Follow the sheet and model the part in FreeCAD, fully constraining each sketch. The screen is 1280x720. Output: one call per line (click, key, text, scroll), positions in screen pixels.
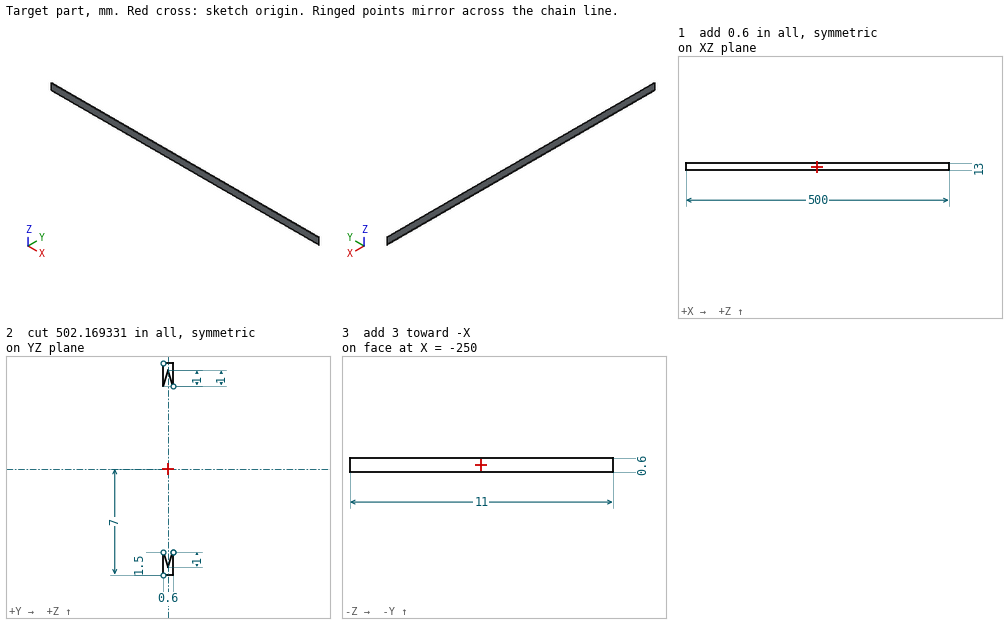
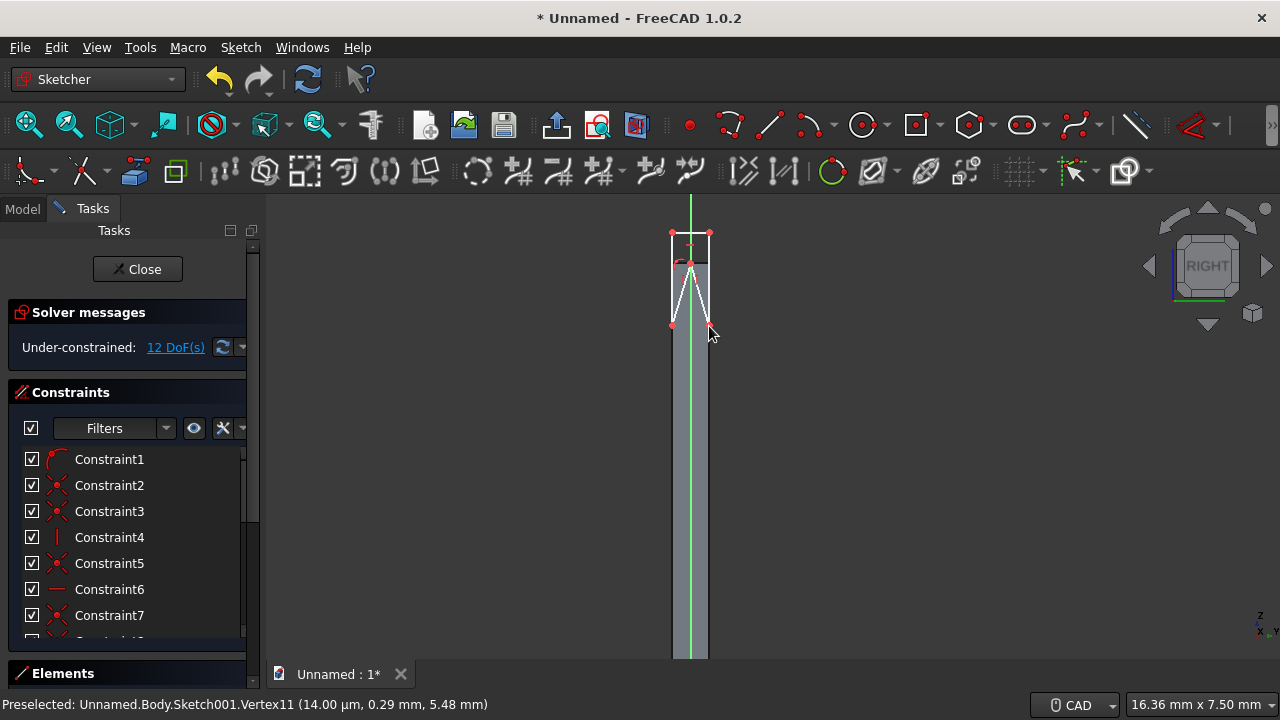
scroll(710, 323, down, 6)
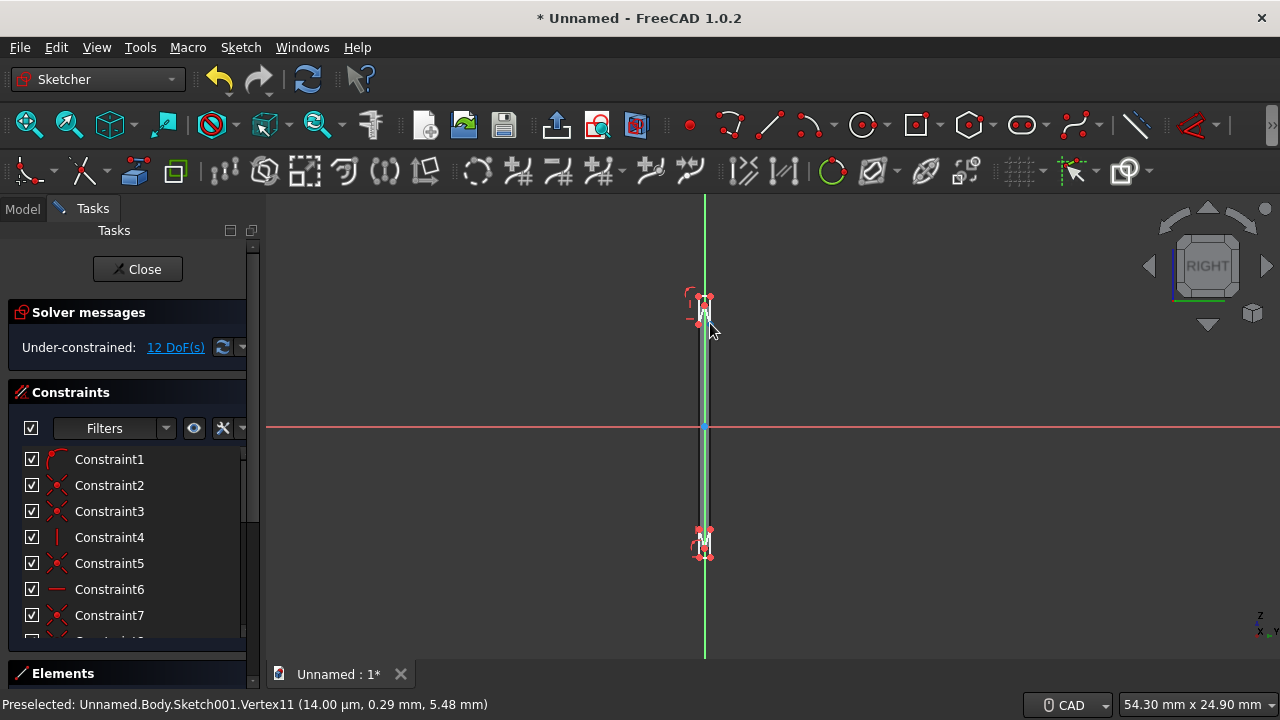
click(710, 530)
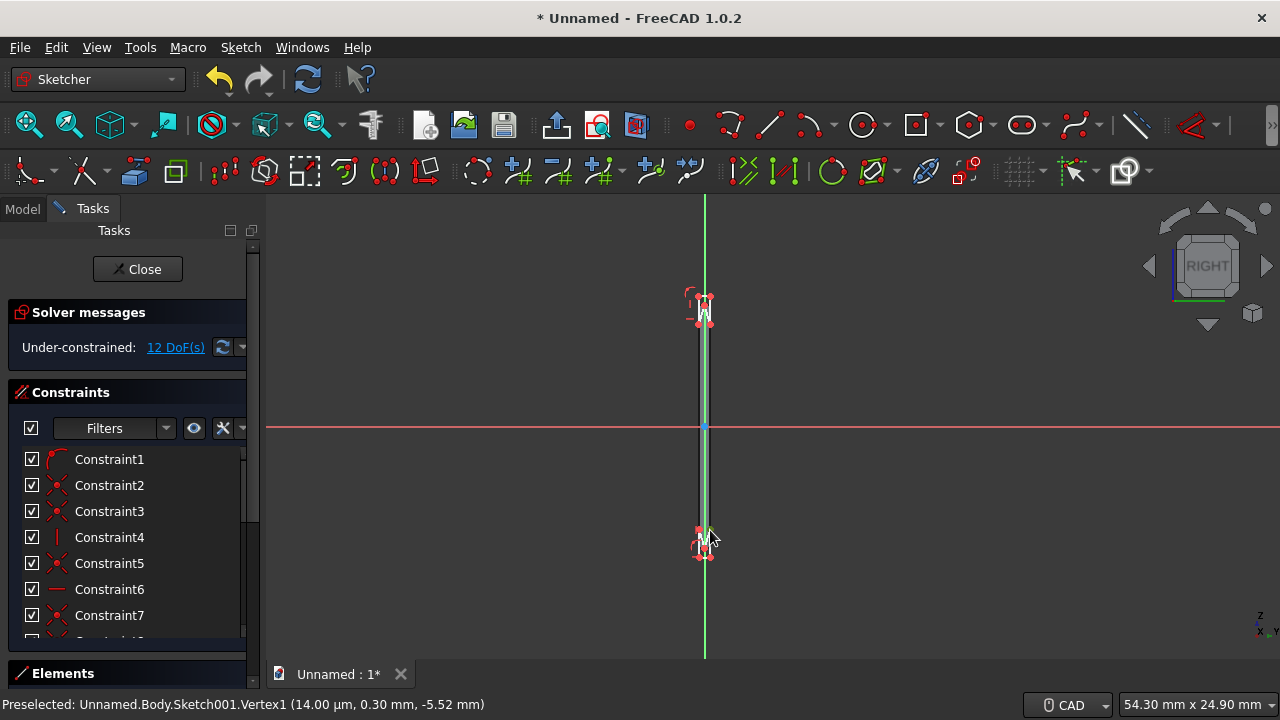
click(699, 530)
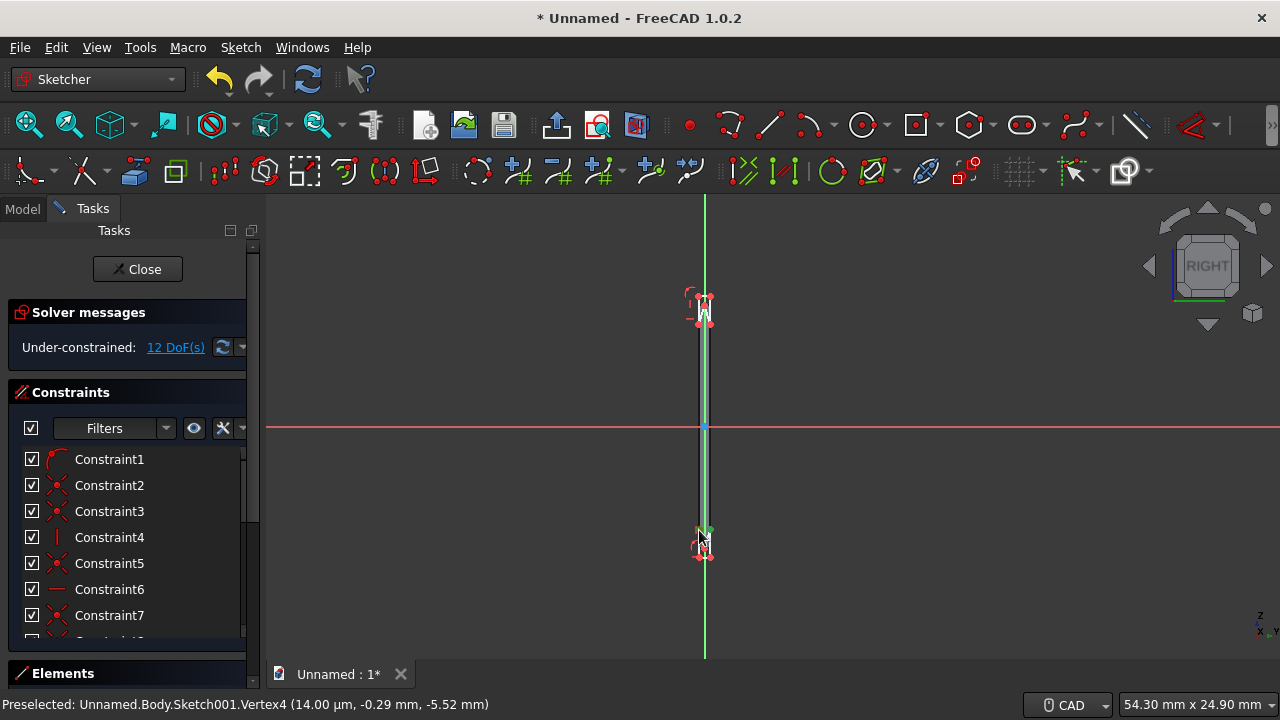
click(705, 602)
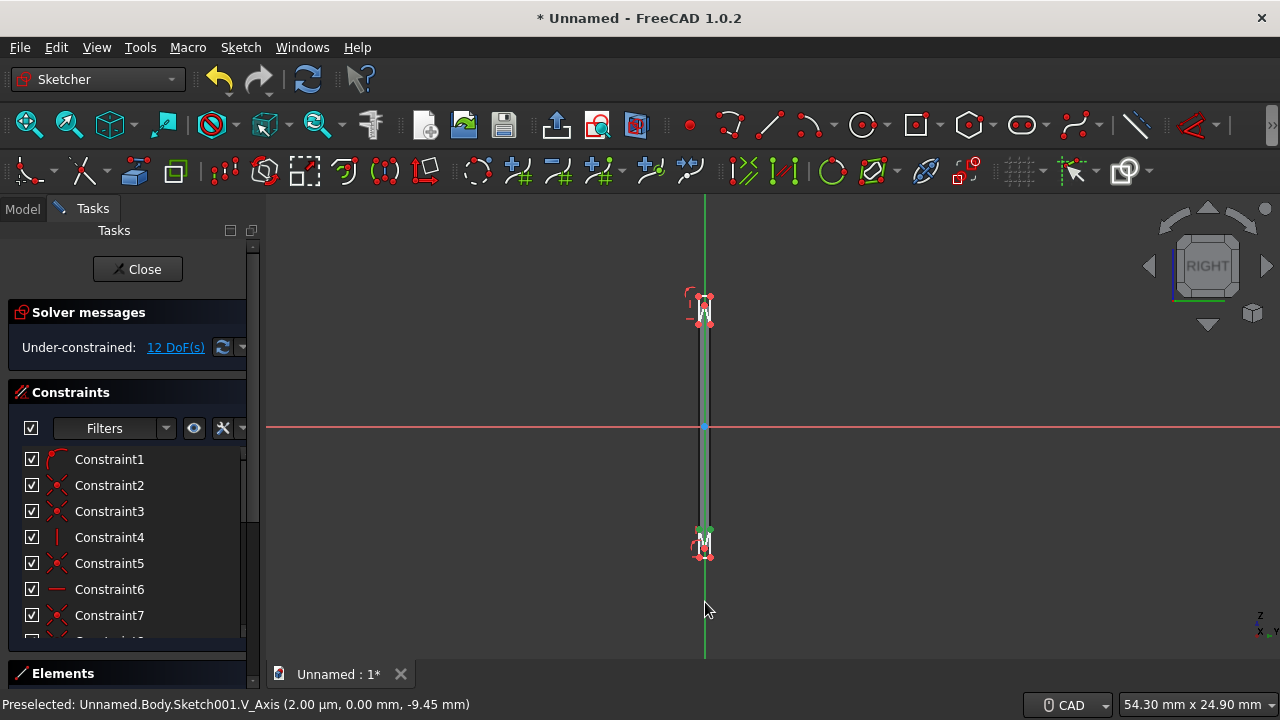
key(s)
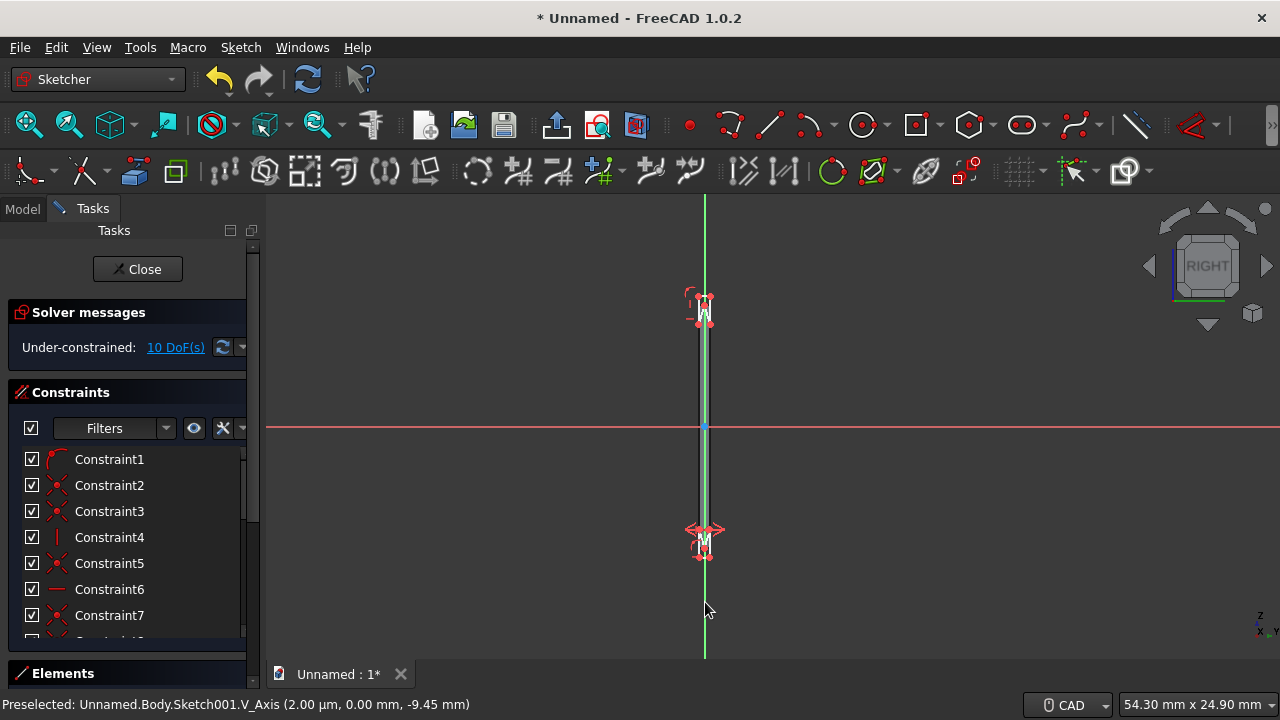
click(710, 530)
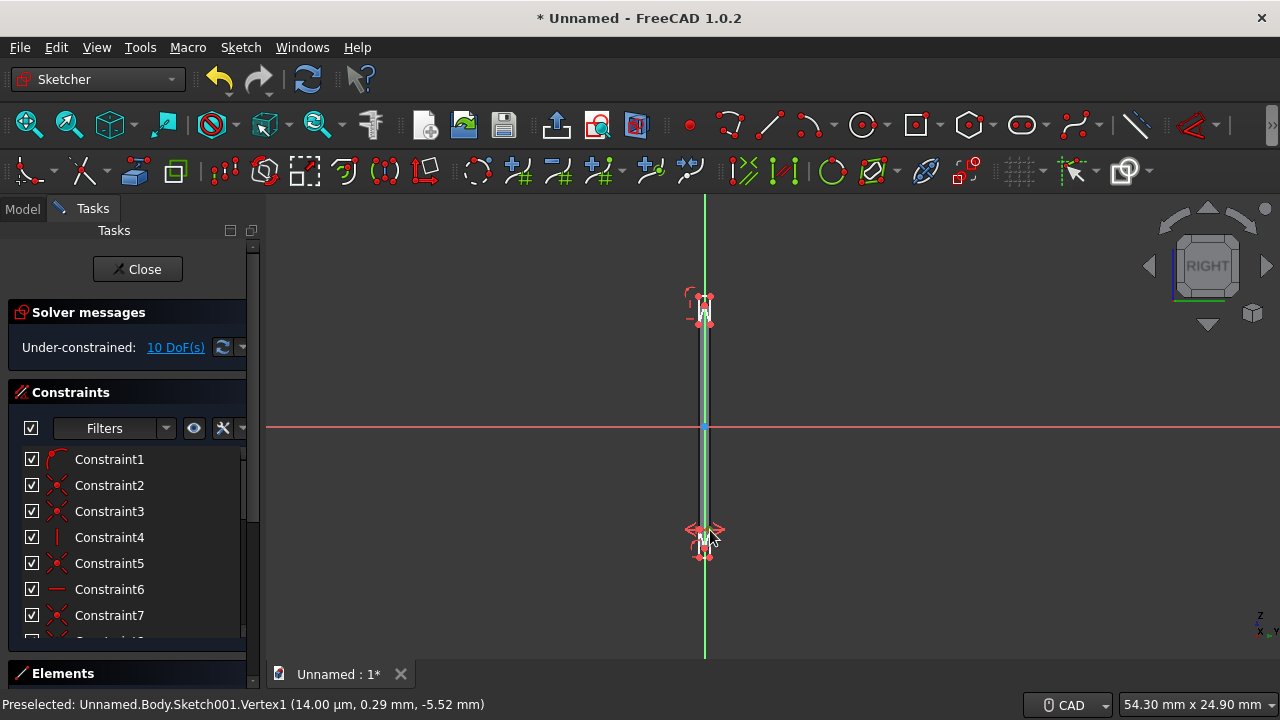
click(710, 324)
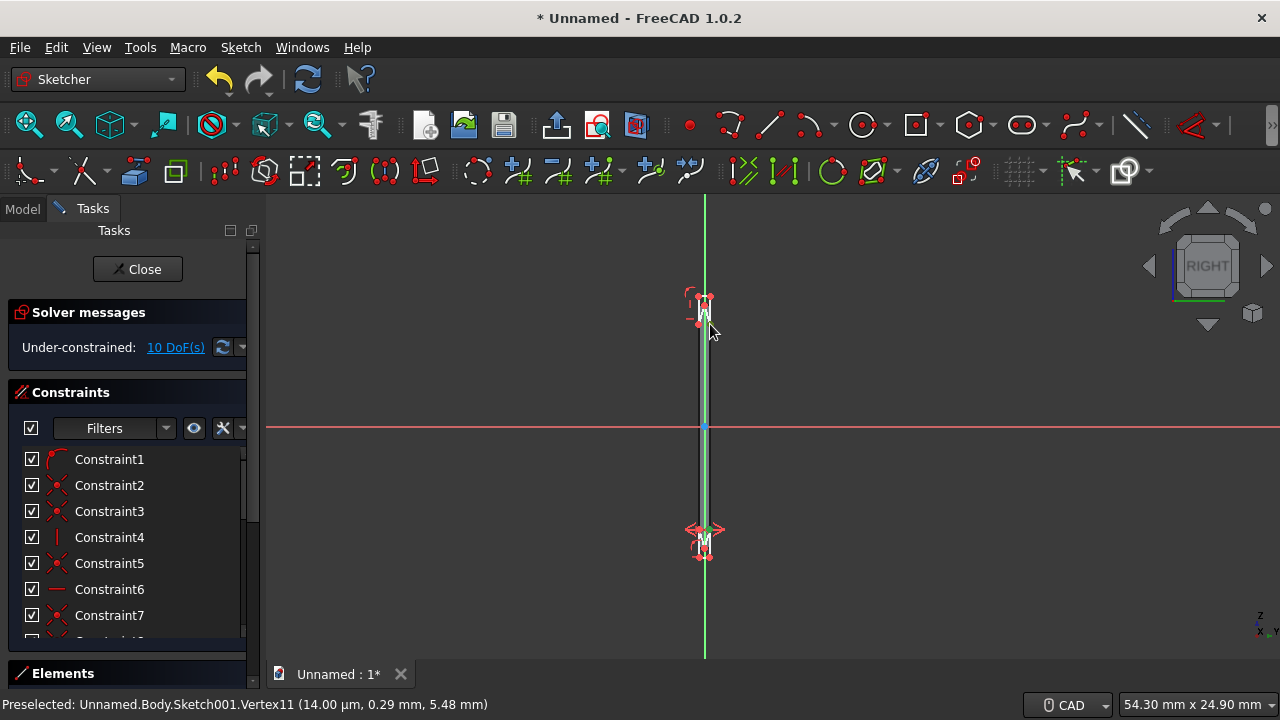
click(353, 426)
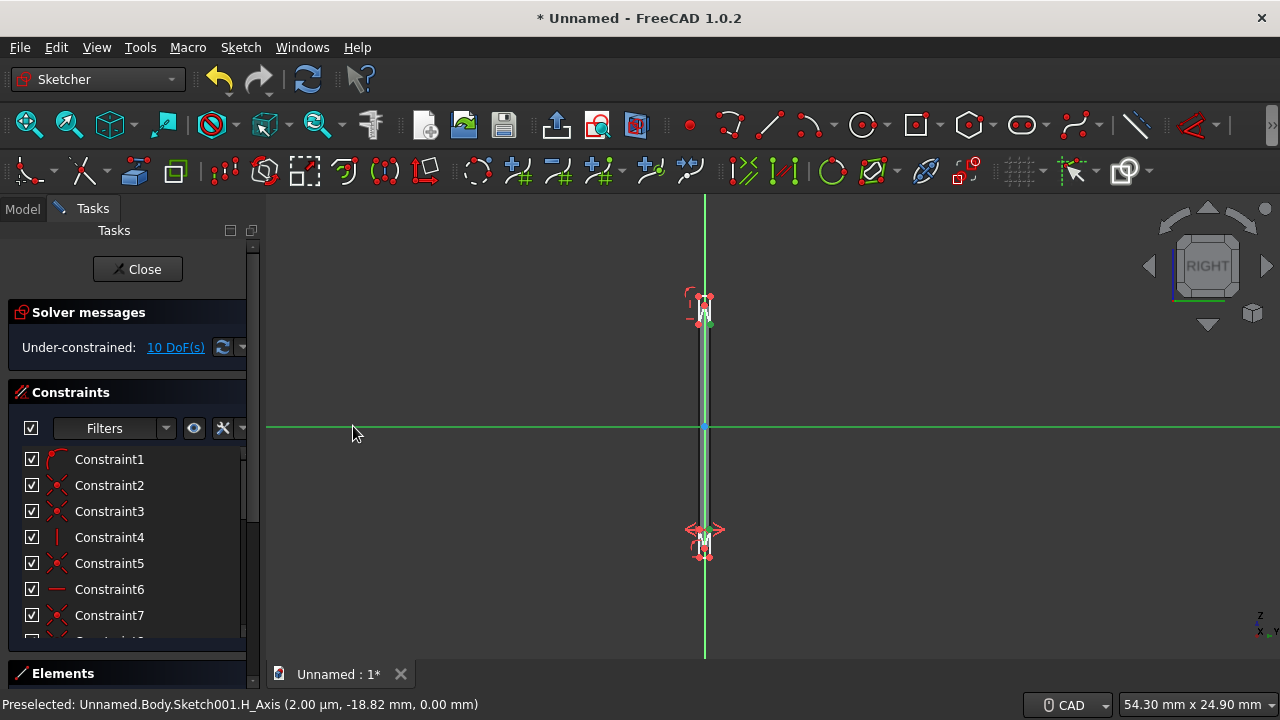
key(s)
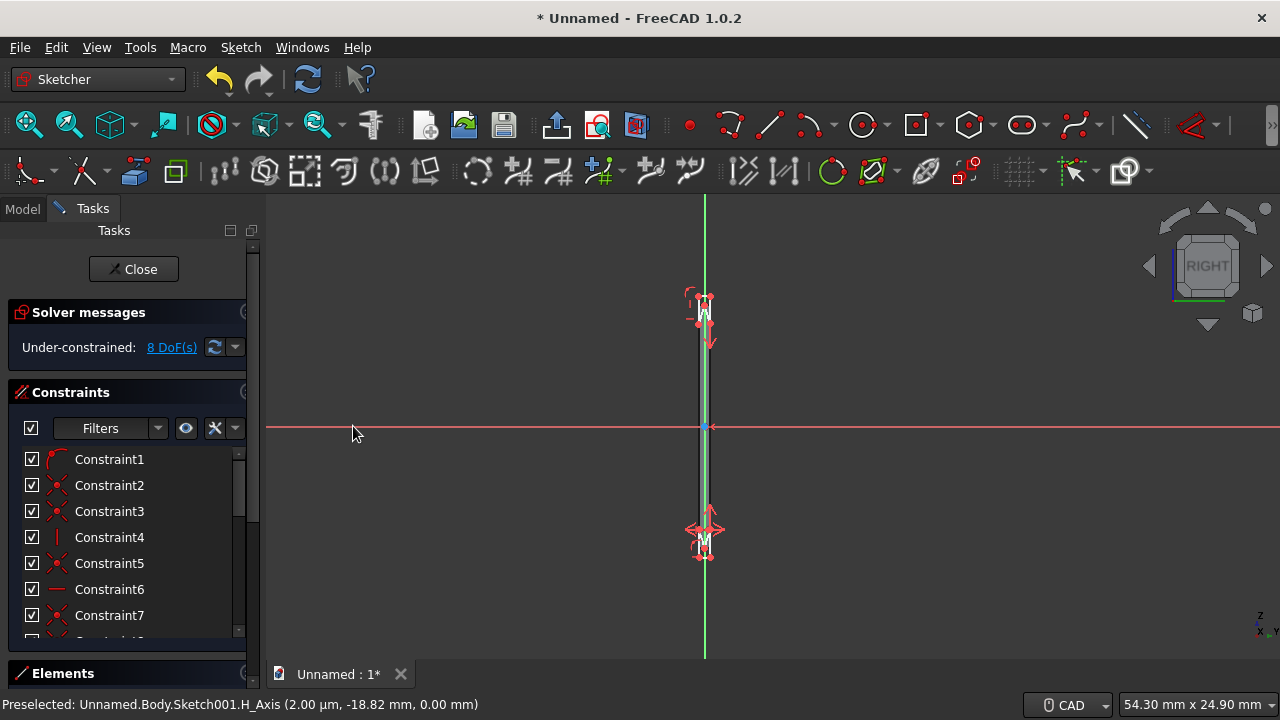
click(699, 558)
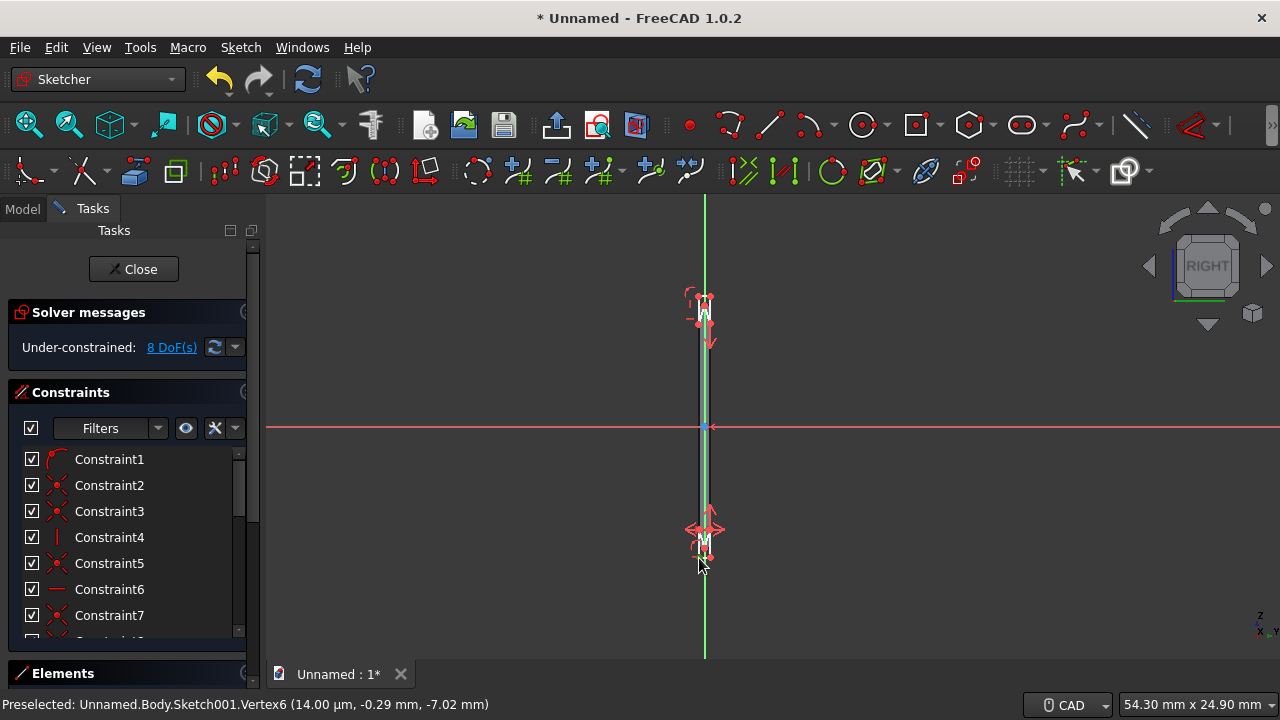
click(699, 296)